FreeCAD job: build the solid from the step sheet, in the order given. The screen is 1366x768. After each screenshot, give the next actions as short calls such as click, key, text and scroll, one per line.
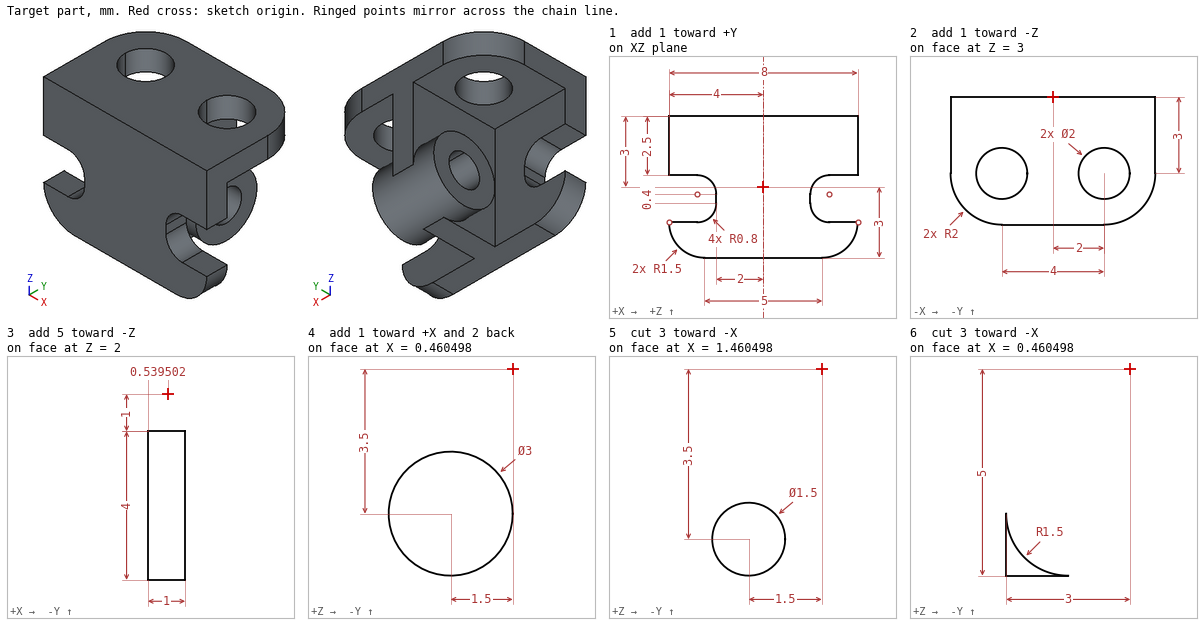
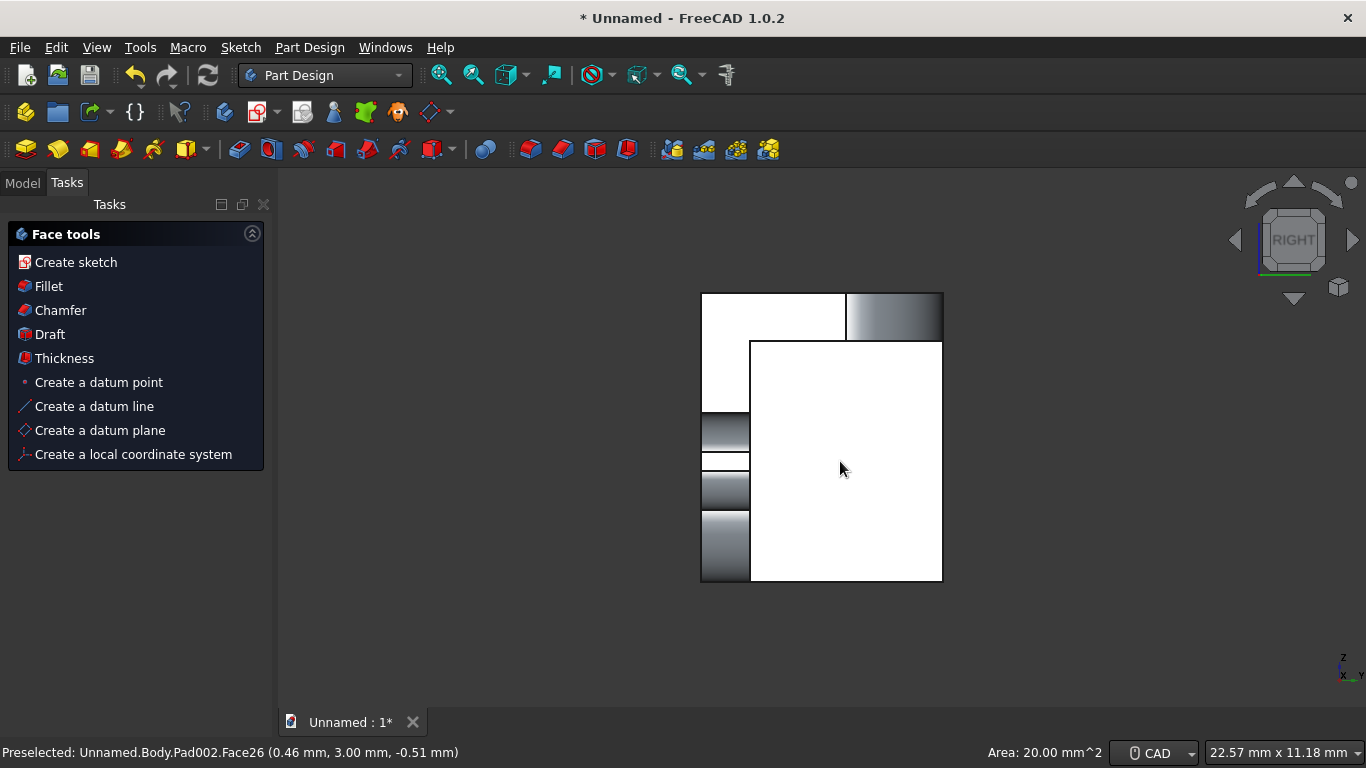
click(258, 112)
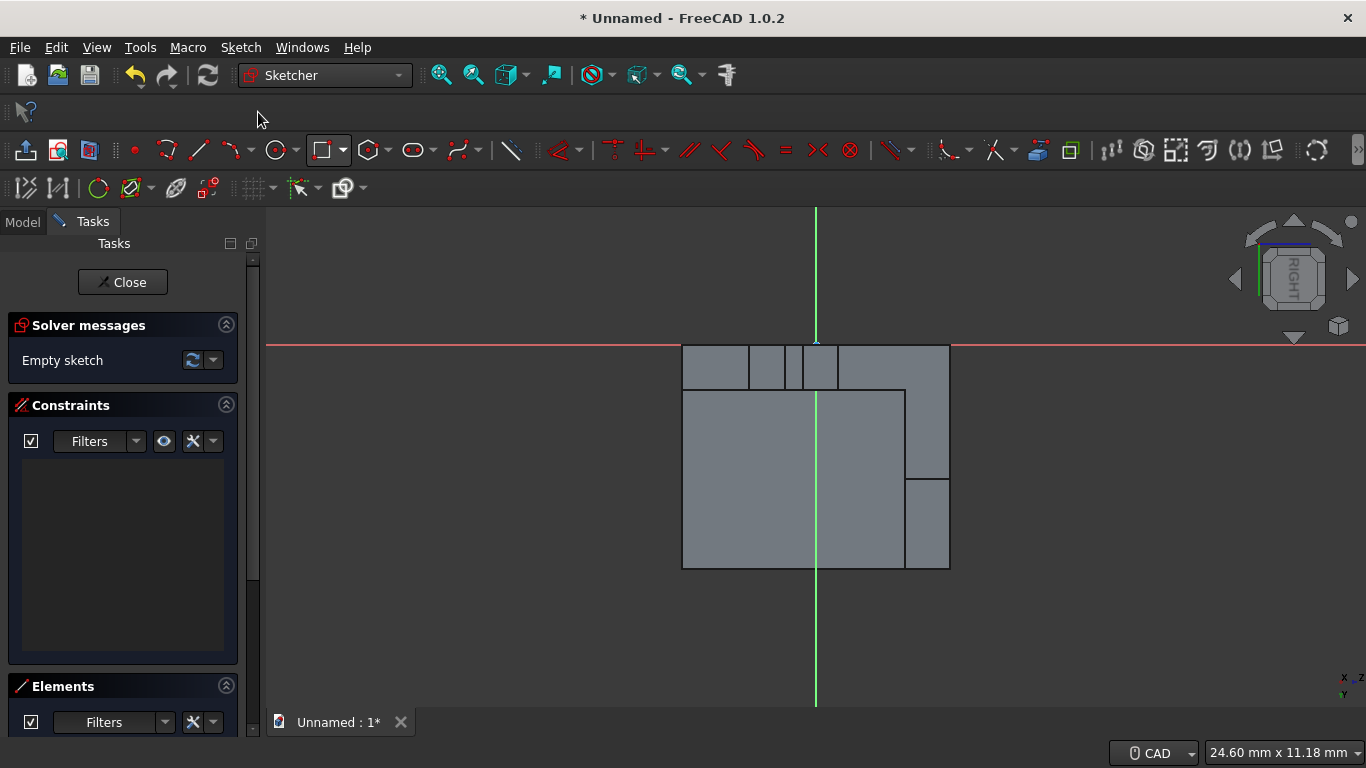
click(90, 150)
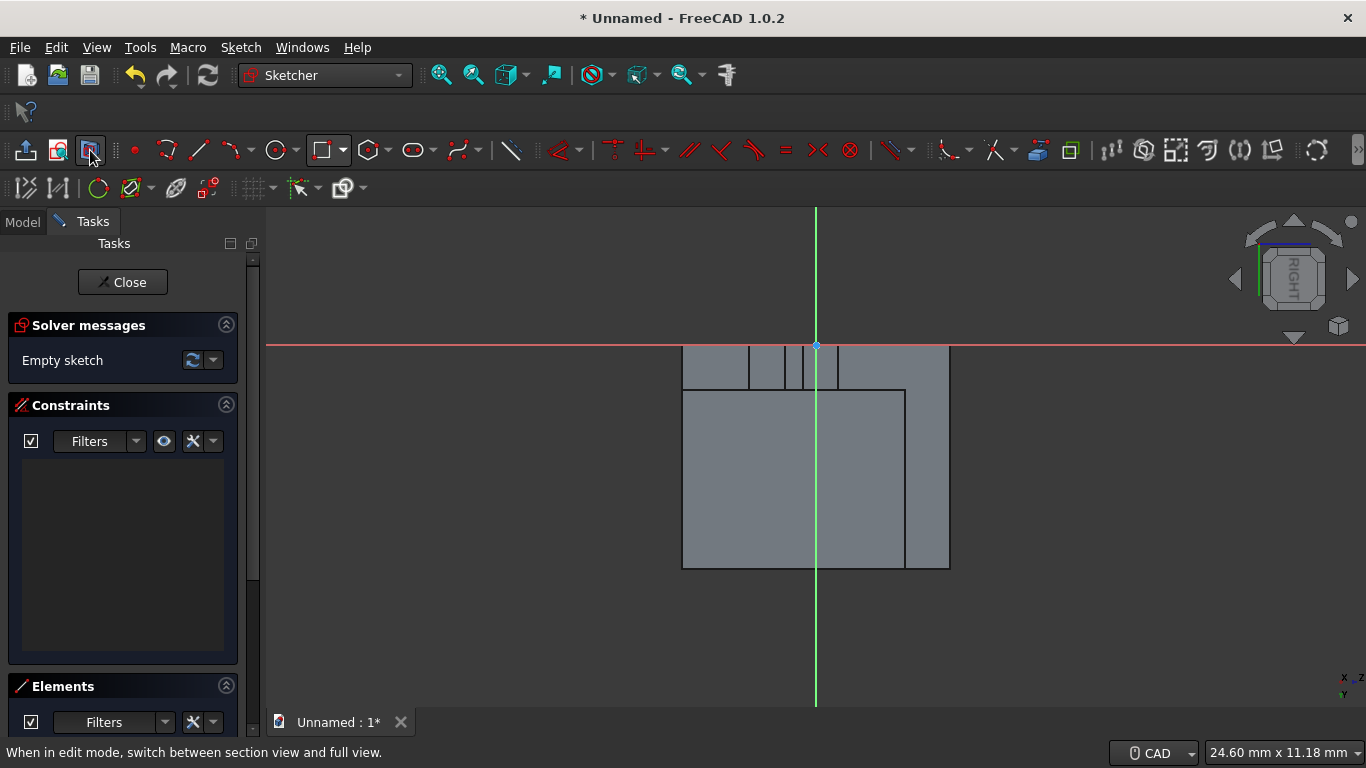
scroll(752, 457, up, 2)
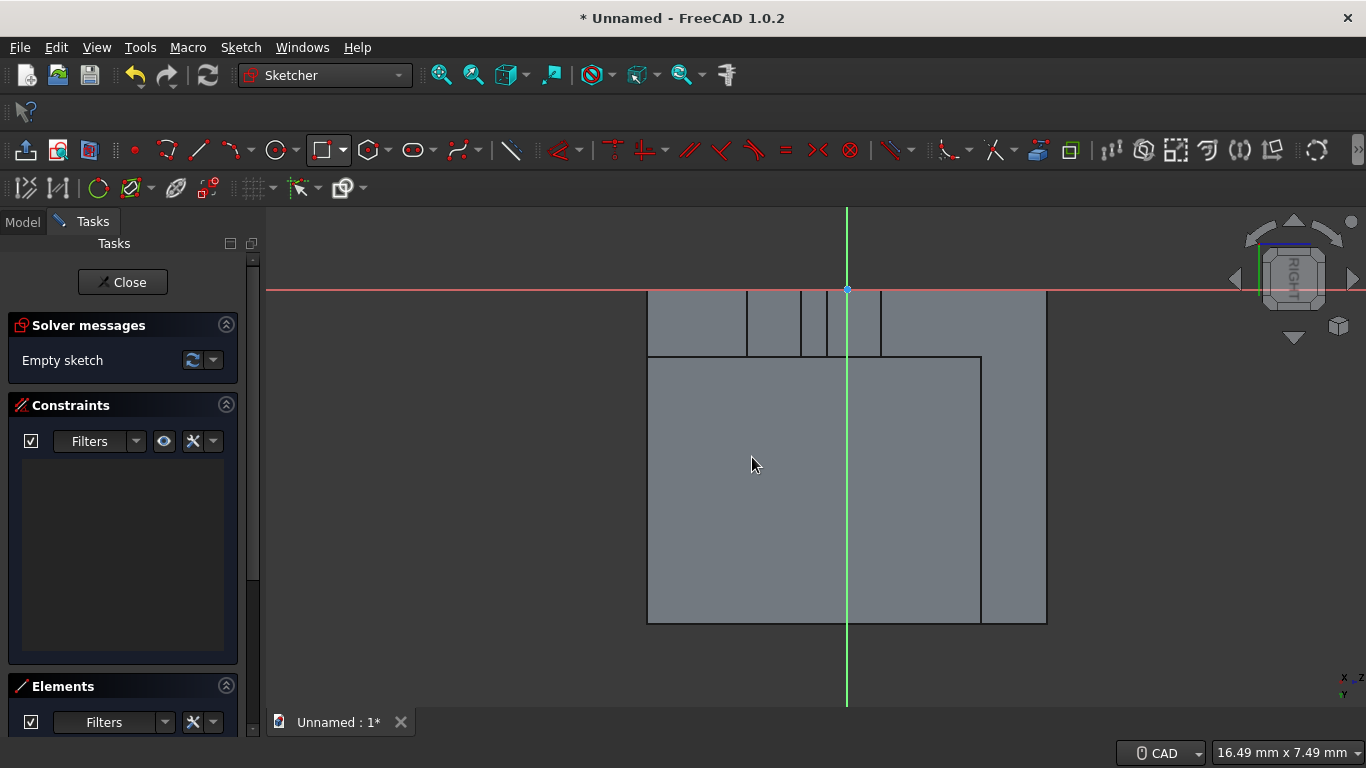
click(276, 150)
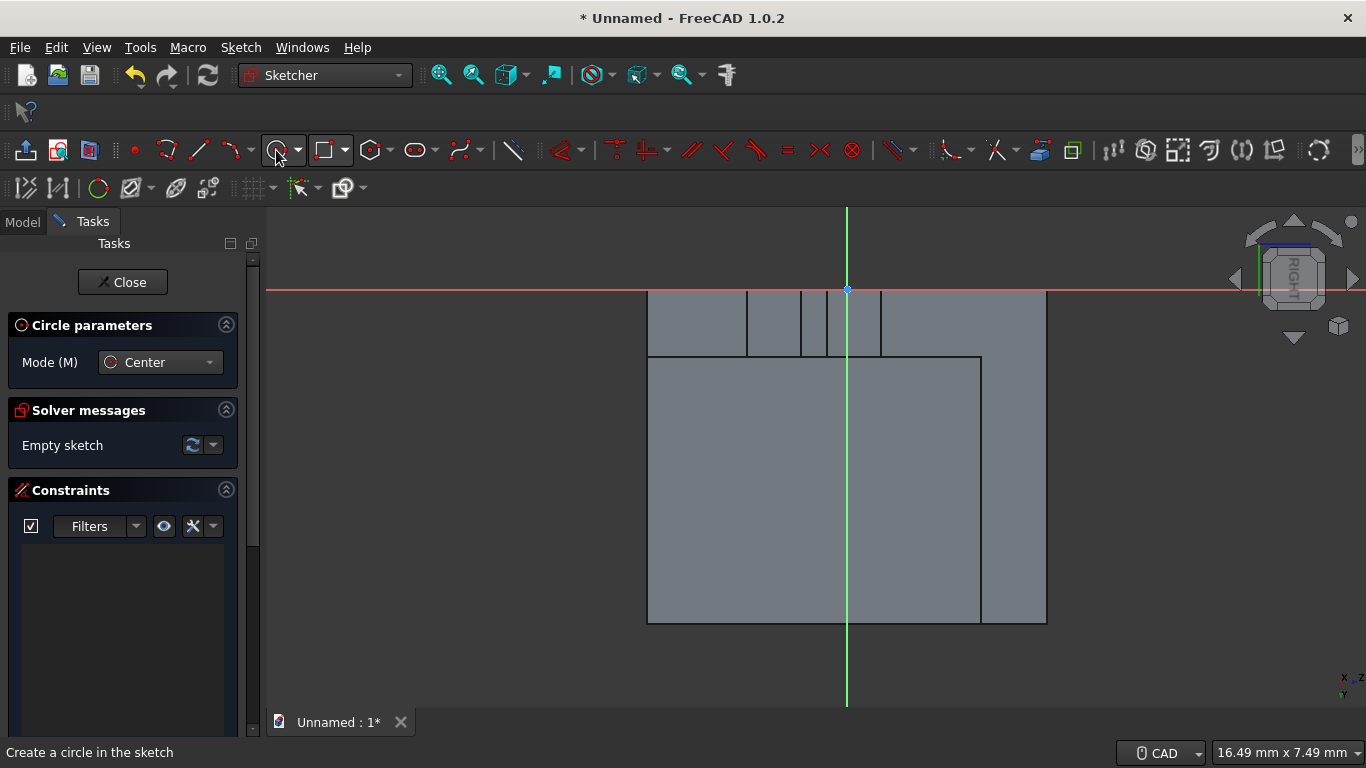
click(747, 523)
click(818, 453)
key(Escape)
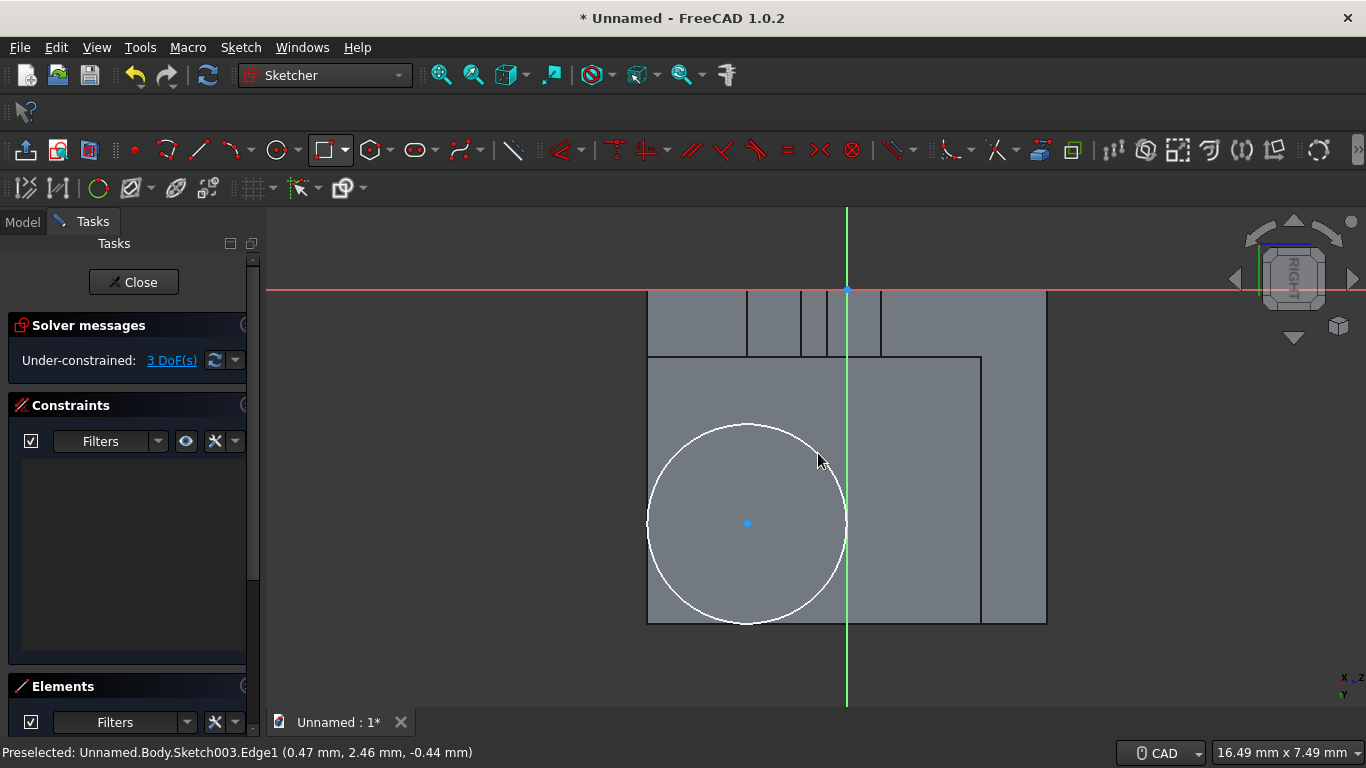
click(560, 150)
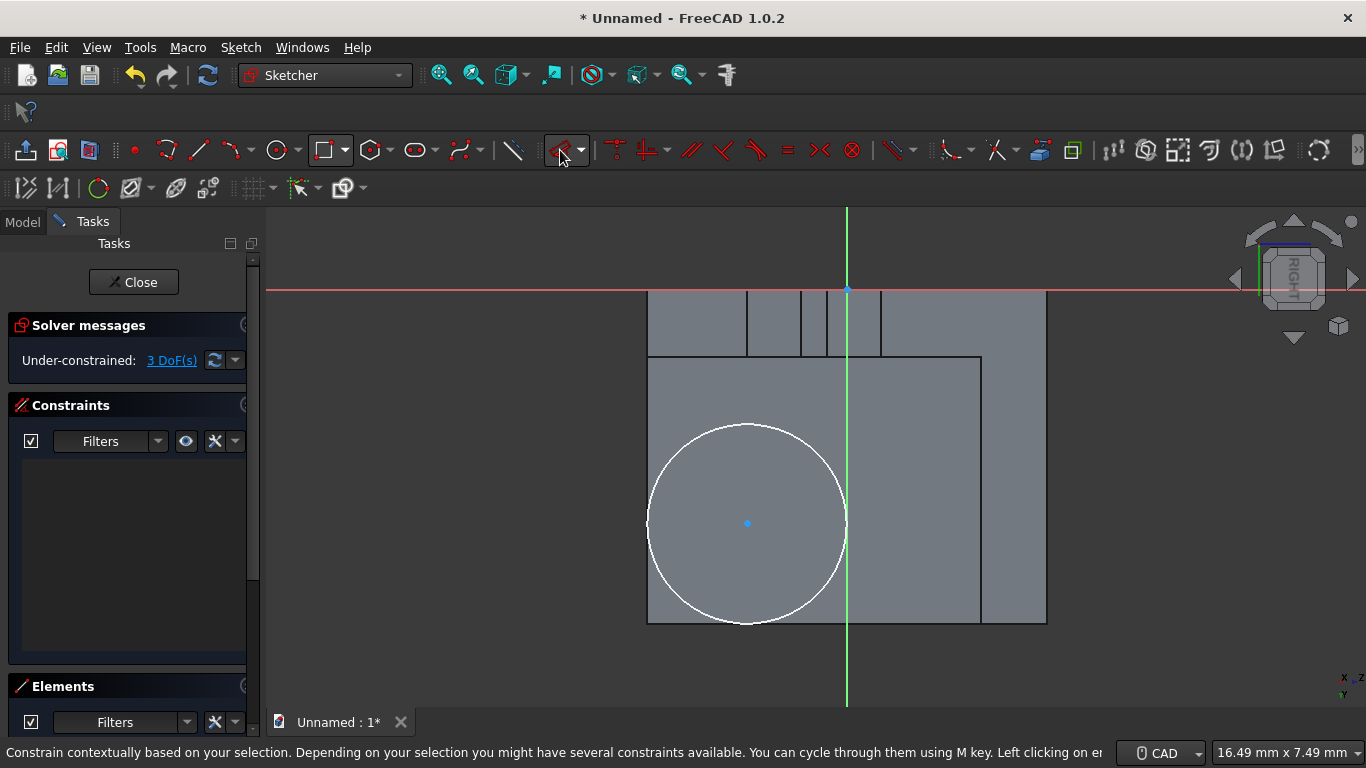
click(817, 453)
click(873, 486)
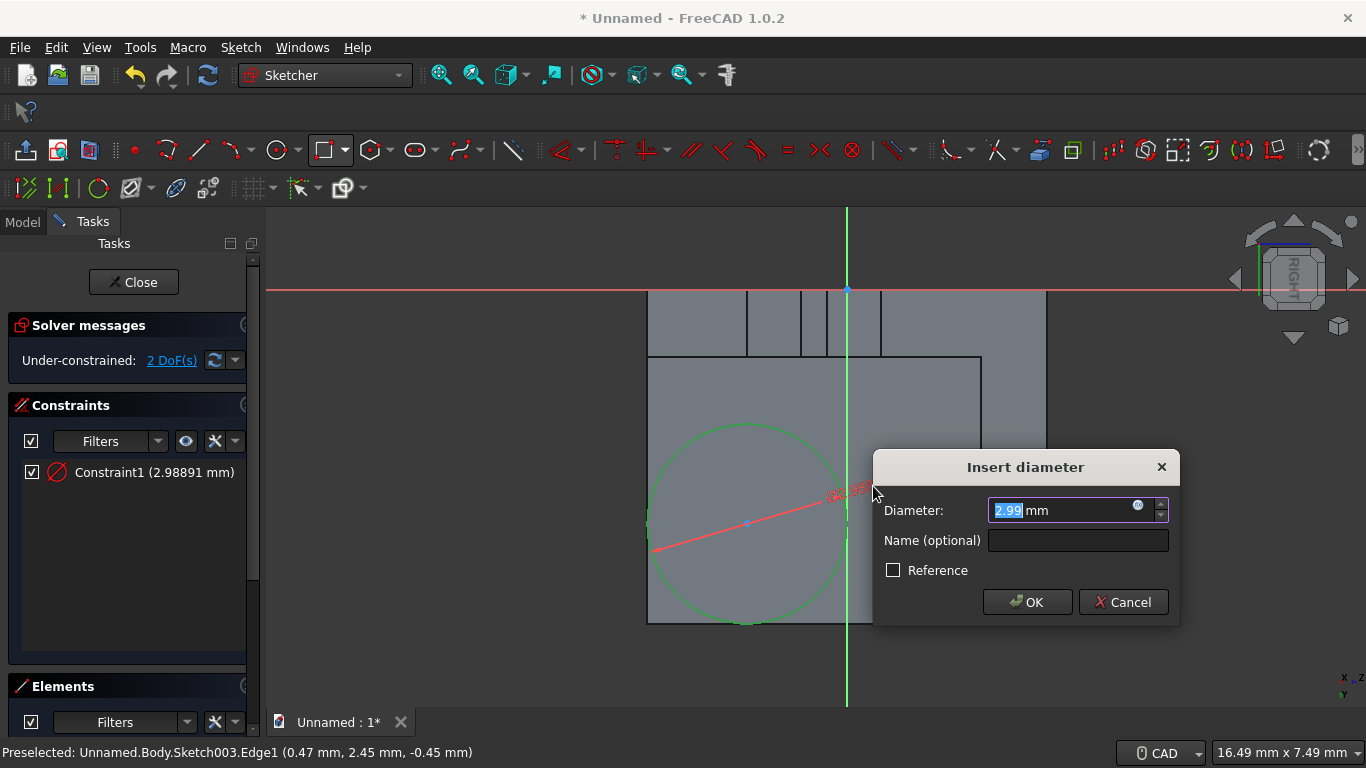
text(3)
key(Return)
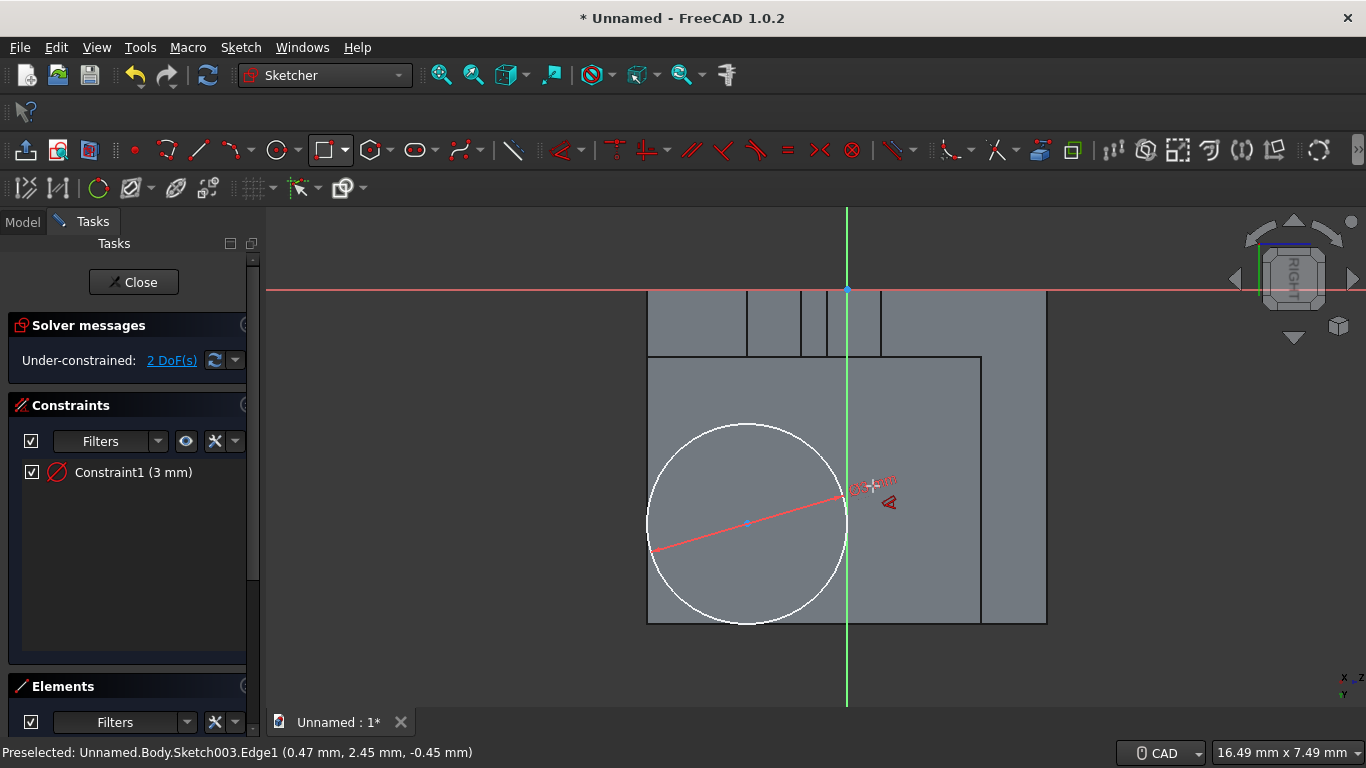
click(747, 524)
click(797, 256)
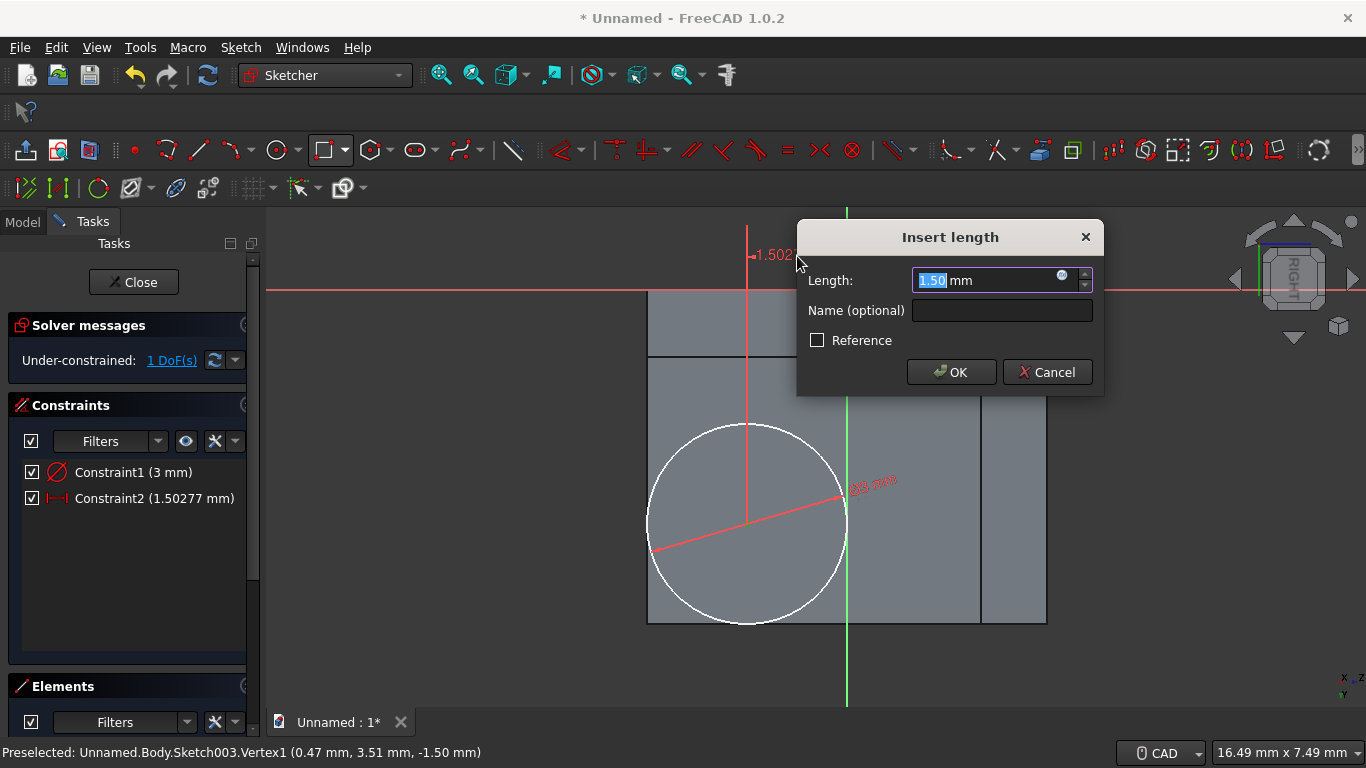
text(1.5)
key(Return)